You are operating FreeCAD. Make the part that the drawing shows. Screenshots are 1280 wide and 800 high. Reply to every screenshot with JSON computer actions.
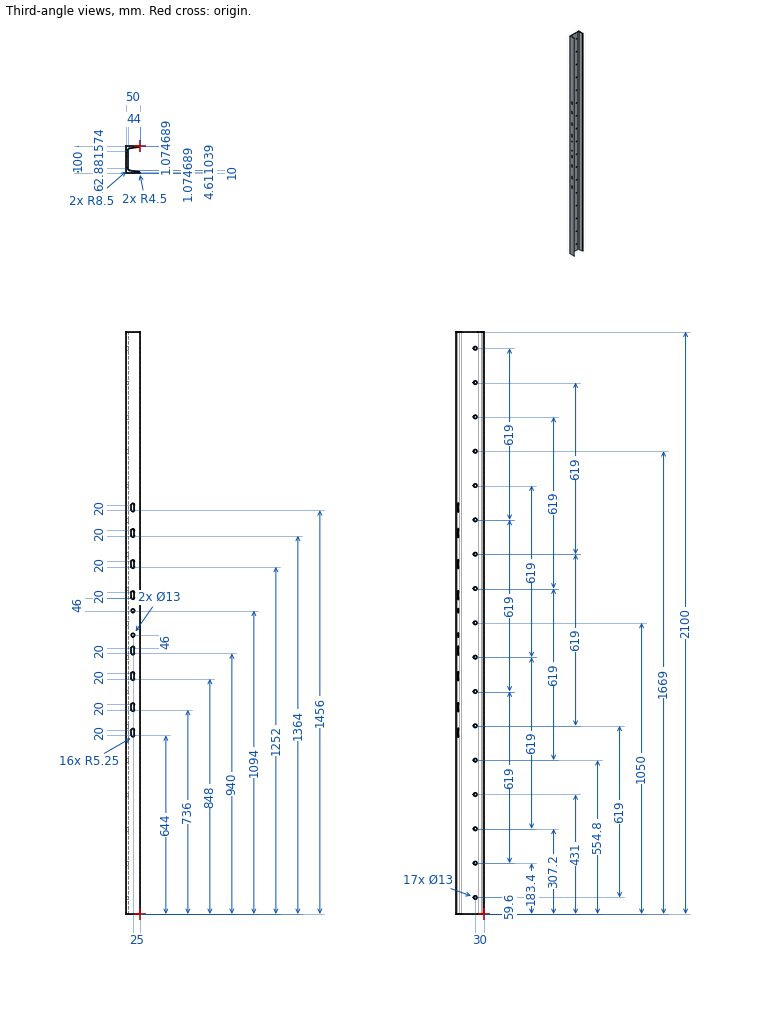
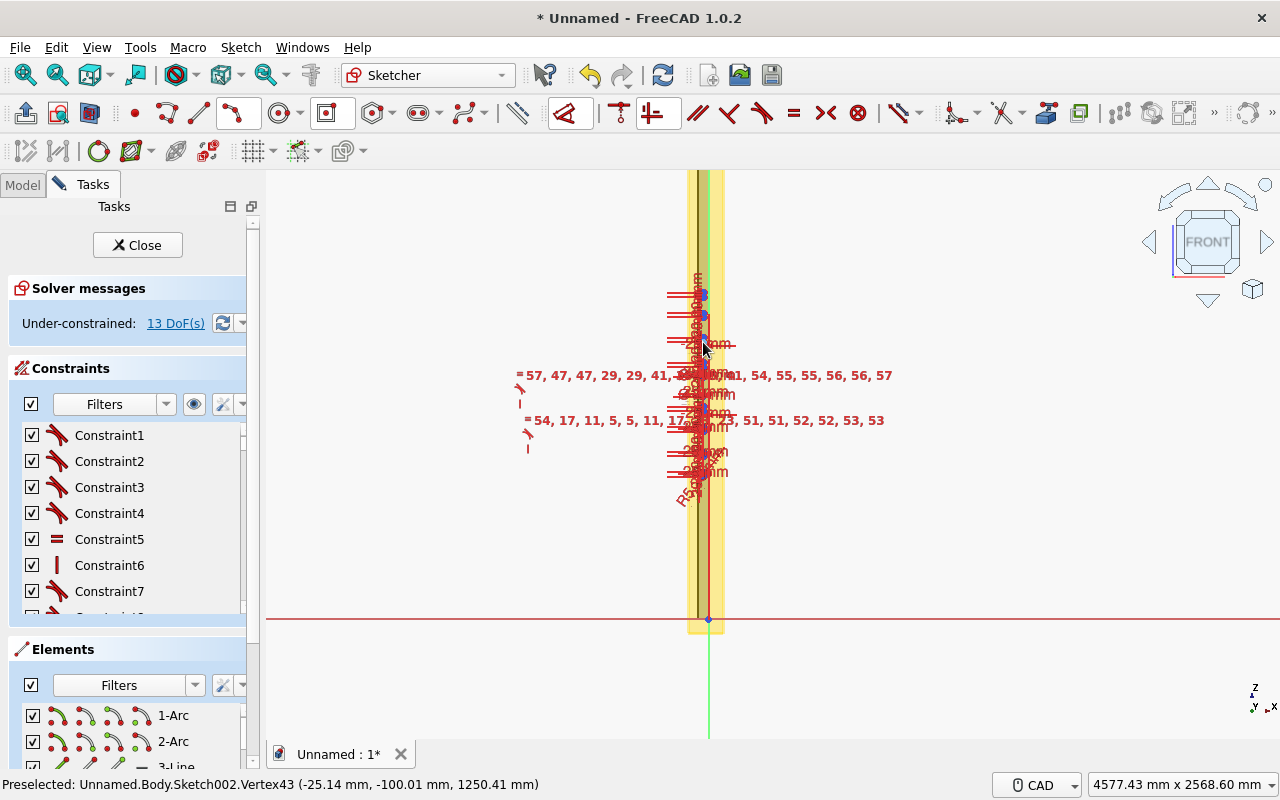
{"action": "scroll", "coordinate": [703, 297], "scroll_direction": "up", "scroll_amount": 12}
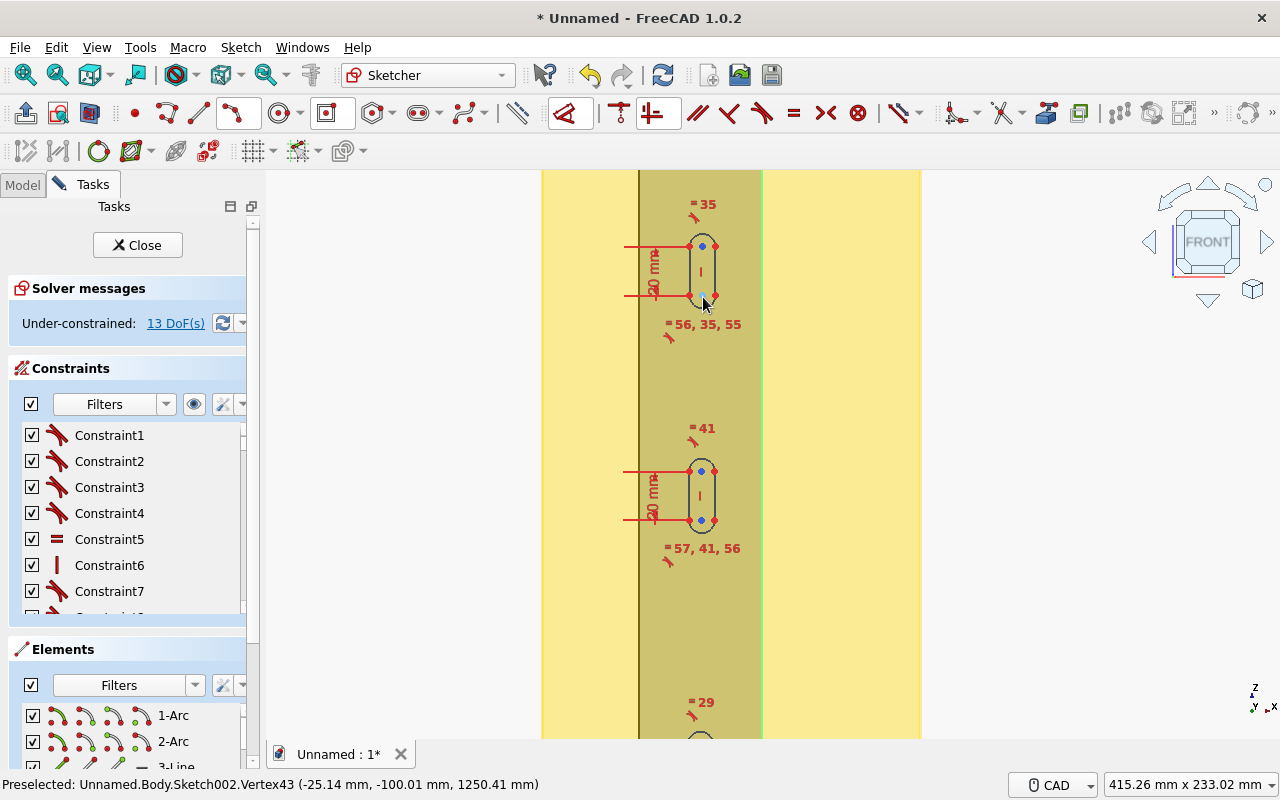
{"action": "left_click", "coordinate": [703, 296]}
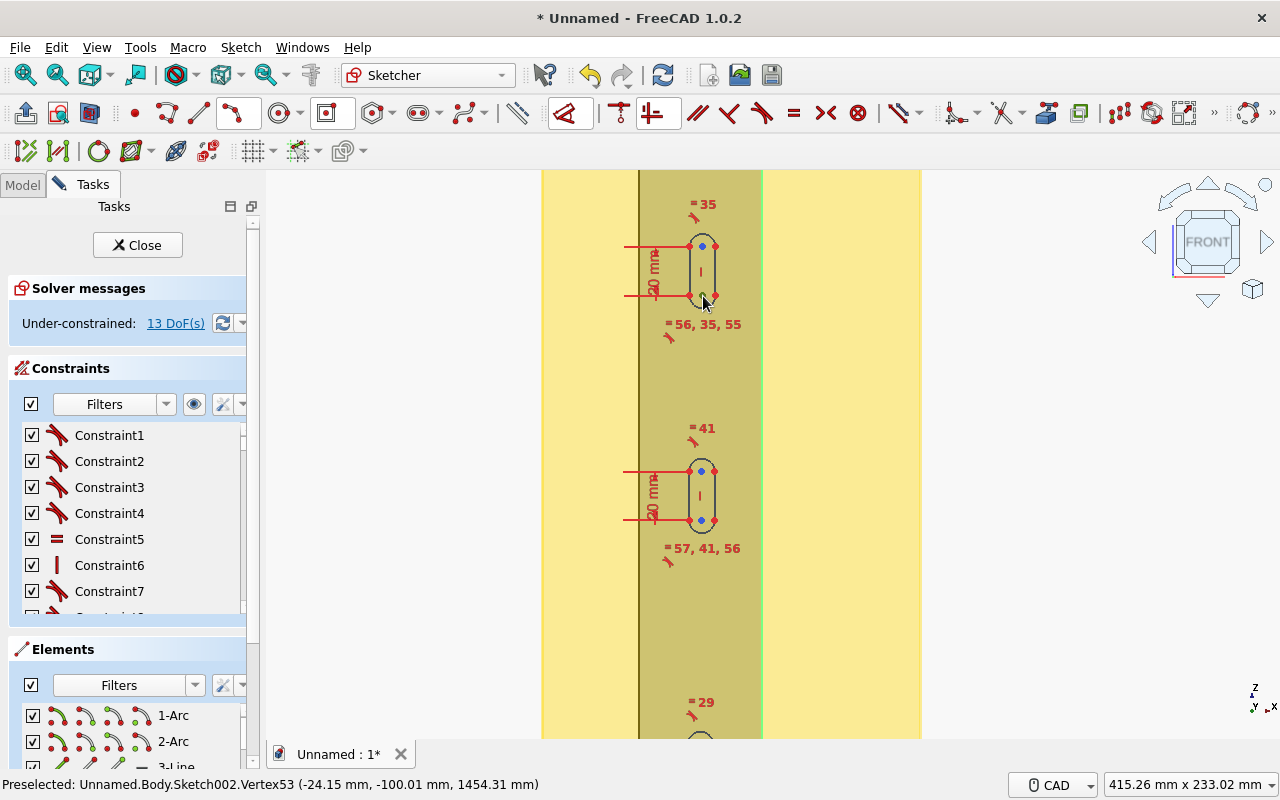
{"action": "key", "text": "l"}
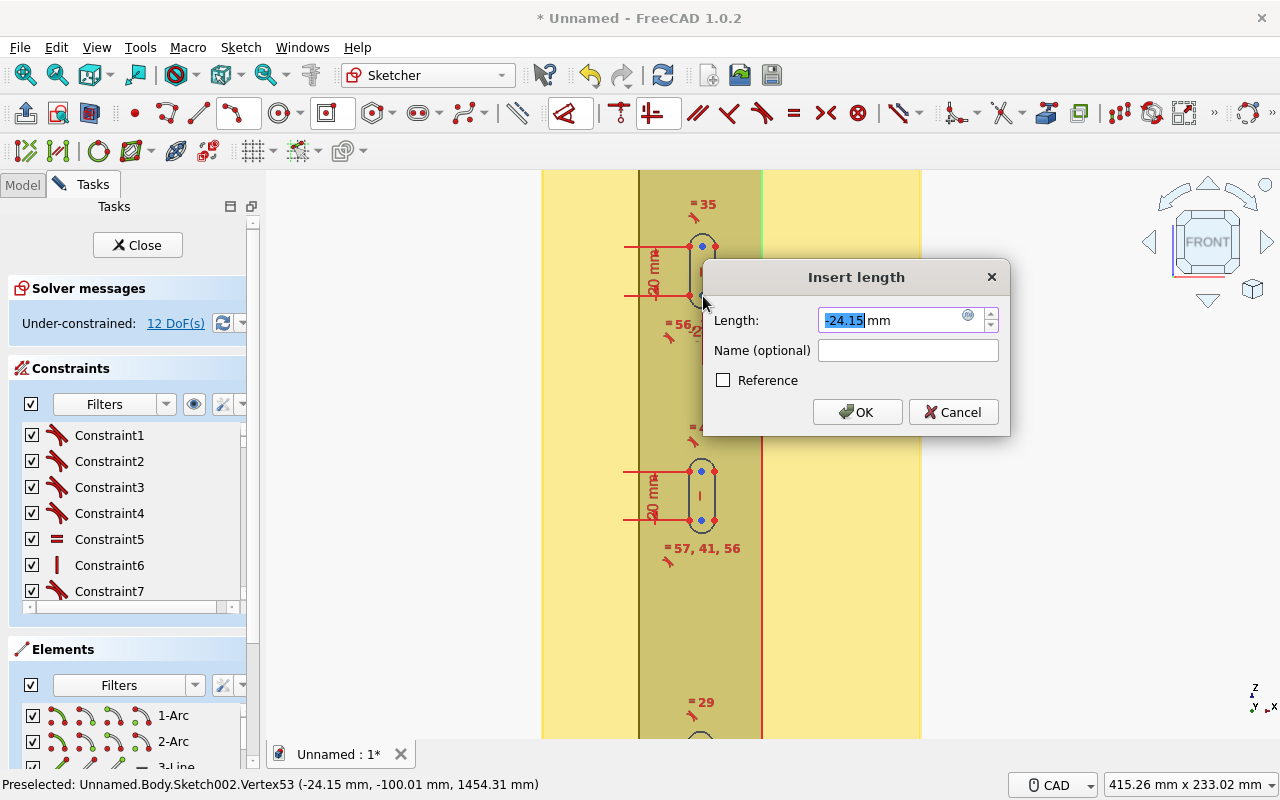
{"action": "type", "text": "-25"}
{"action": "key", "text": "Return"}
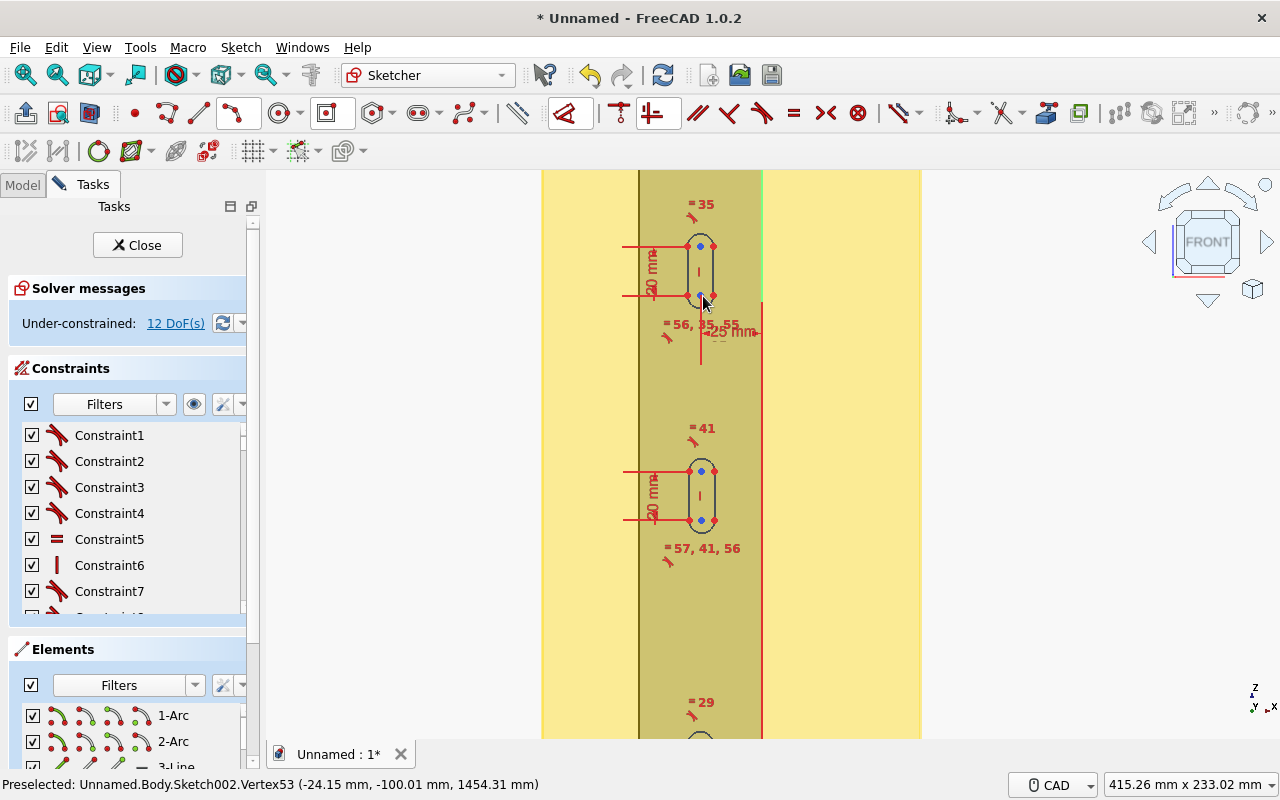
{"action": "left_click", "coordinate": [702, 520]}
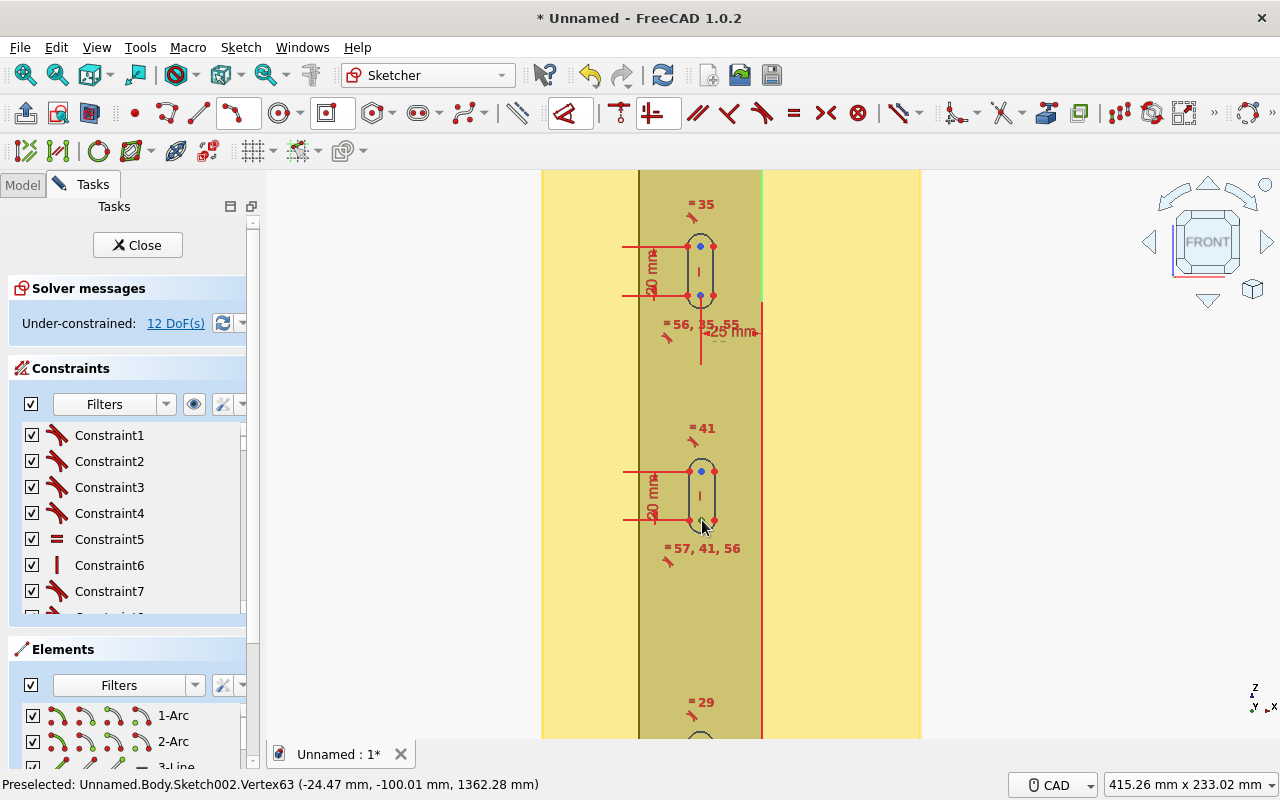
{"action": "key", "text": "l"}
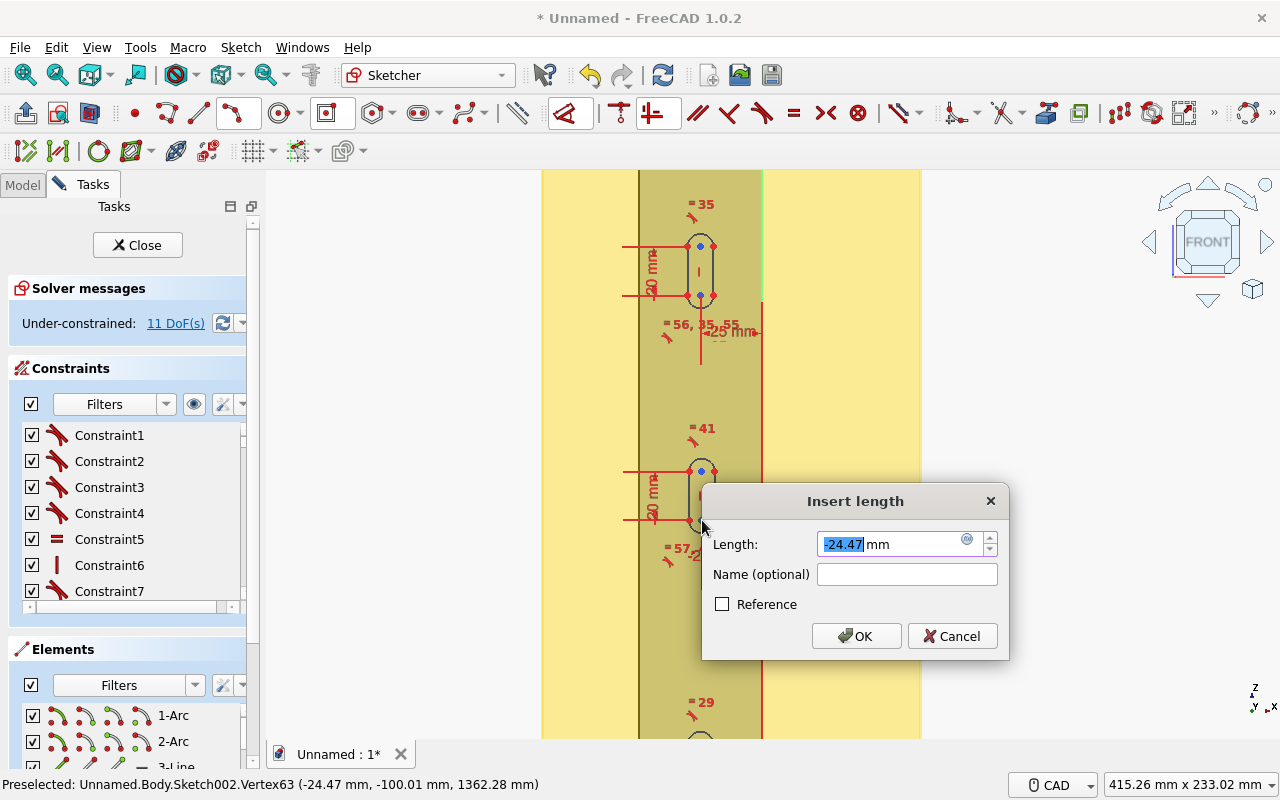
{"action": "type", "text": "-25"}
{"action": "key", "text": "Return"}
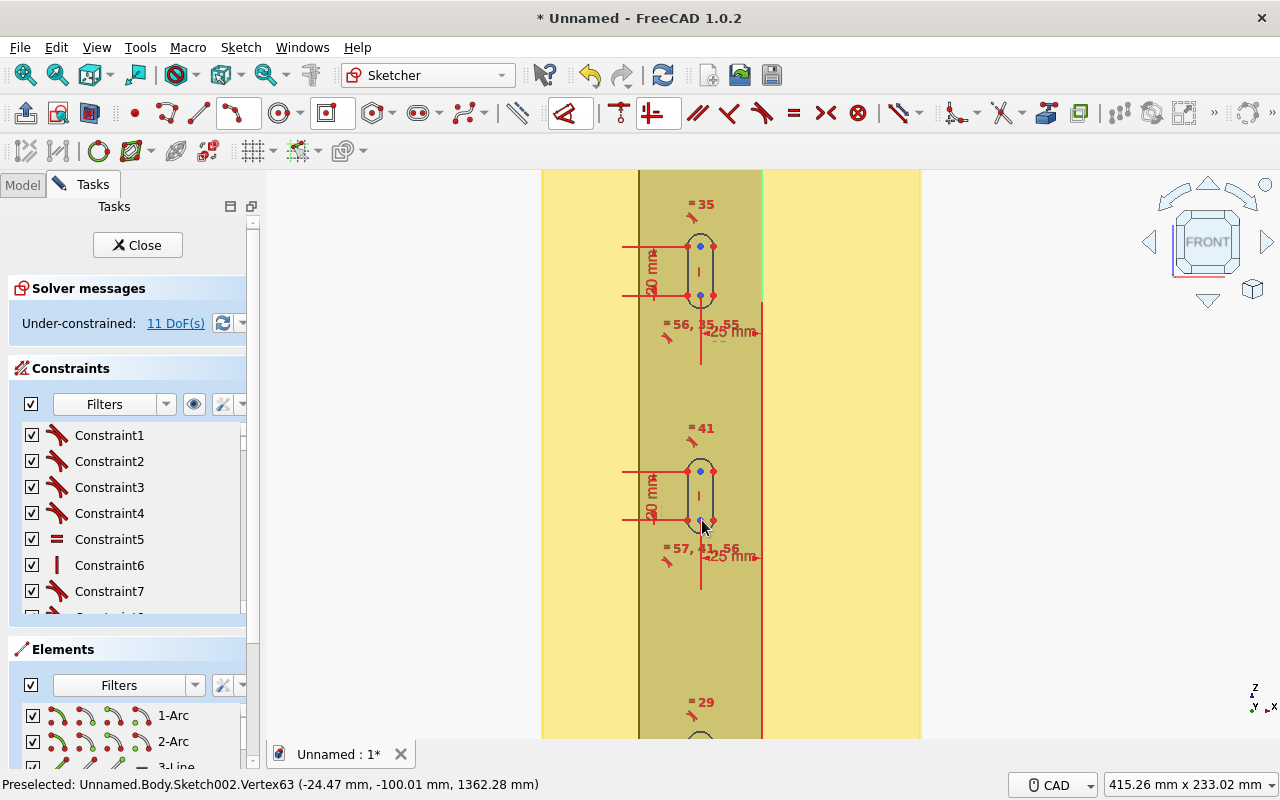
{"action": "scroll", "coordinate": [703, 296], "scroll_direction": "down", "scroll_amount": 12}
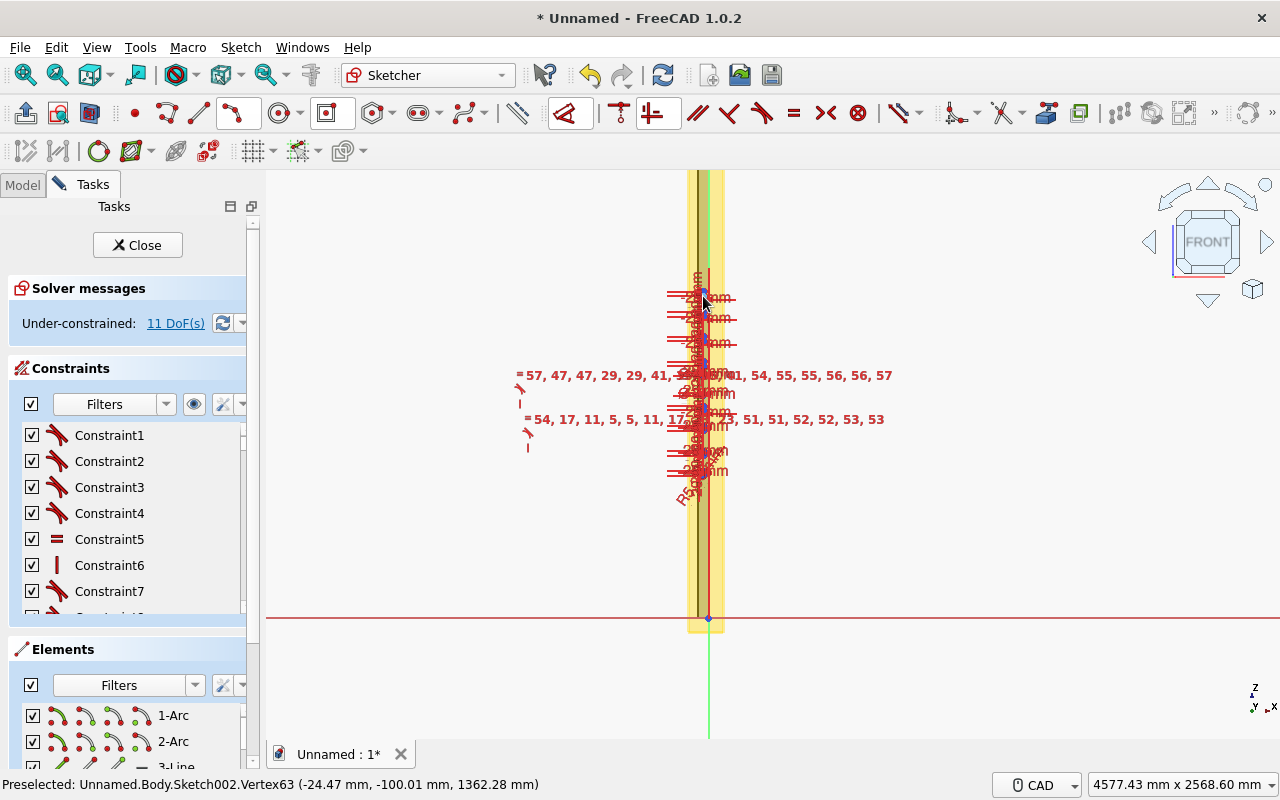
{"action": "scroll", "coordinate": [703, 366], "scroll_direction": "up", "scroll_amount": 12}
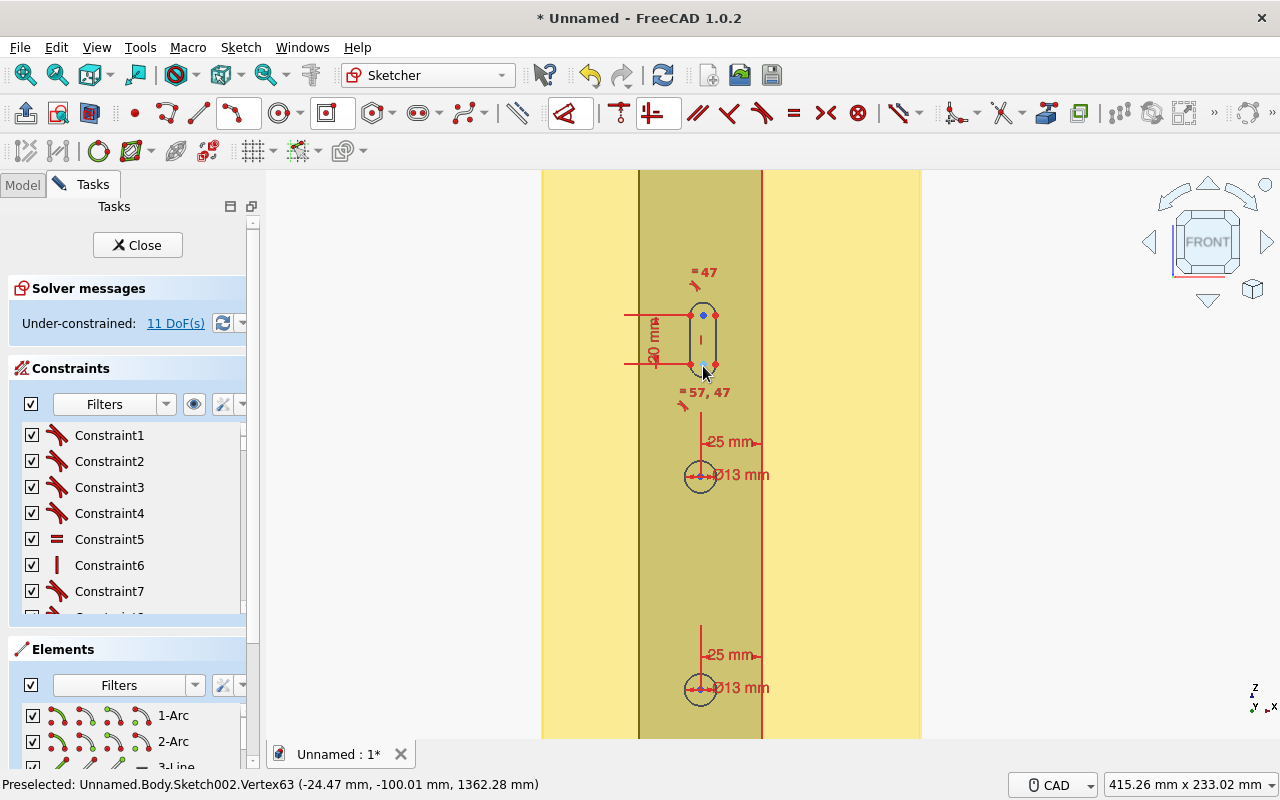
{"action": "left_click", "coordinate": [703, 364]}